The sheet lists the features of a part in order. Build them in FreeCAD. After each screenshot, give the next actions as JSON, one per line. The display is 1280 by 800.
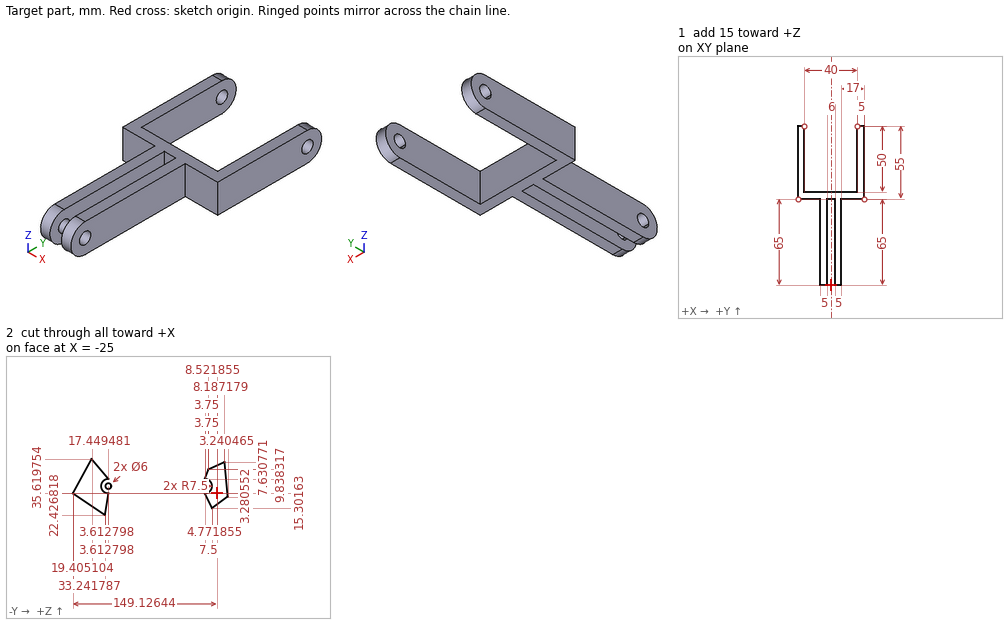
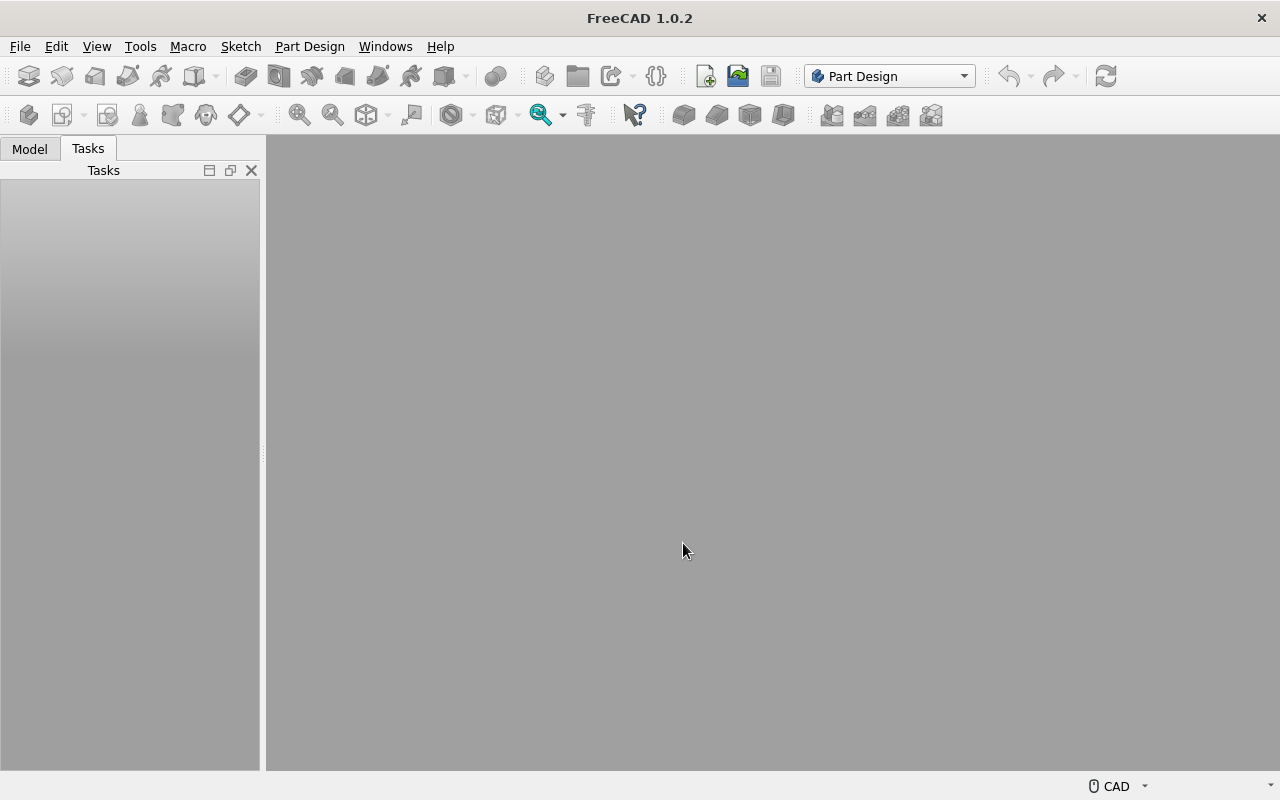
{"action": "key", "text": "ctrl+n"}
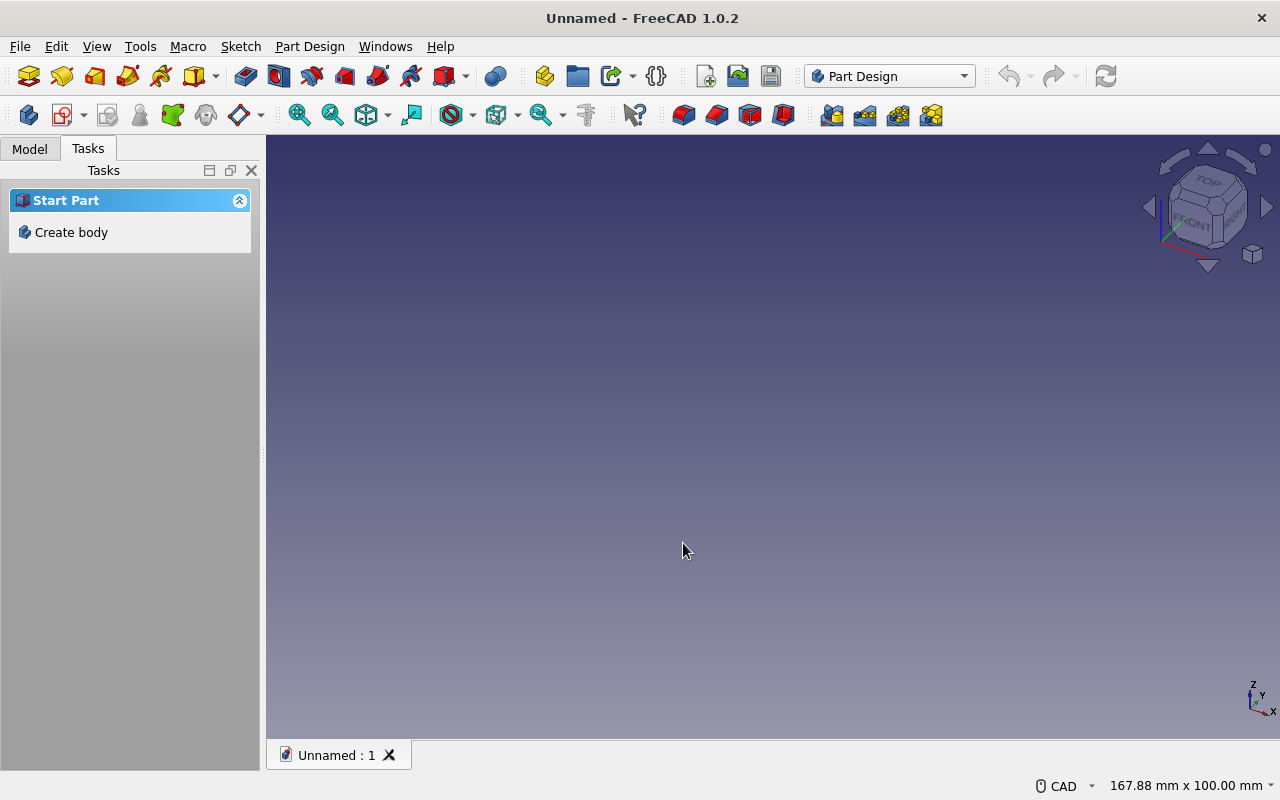
{"action": "left_click", "coordinate": [62, 116]}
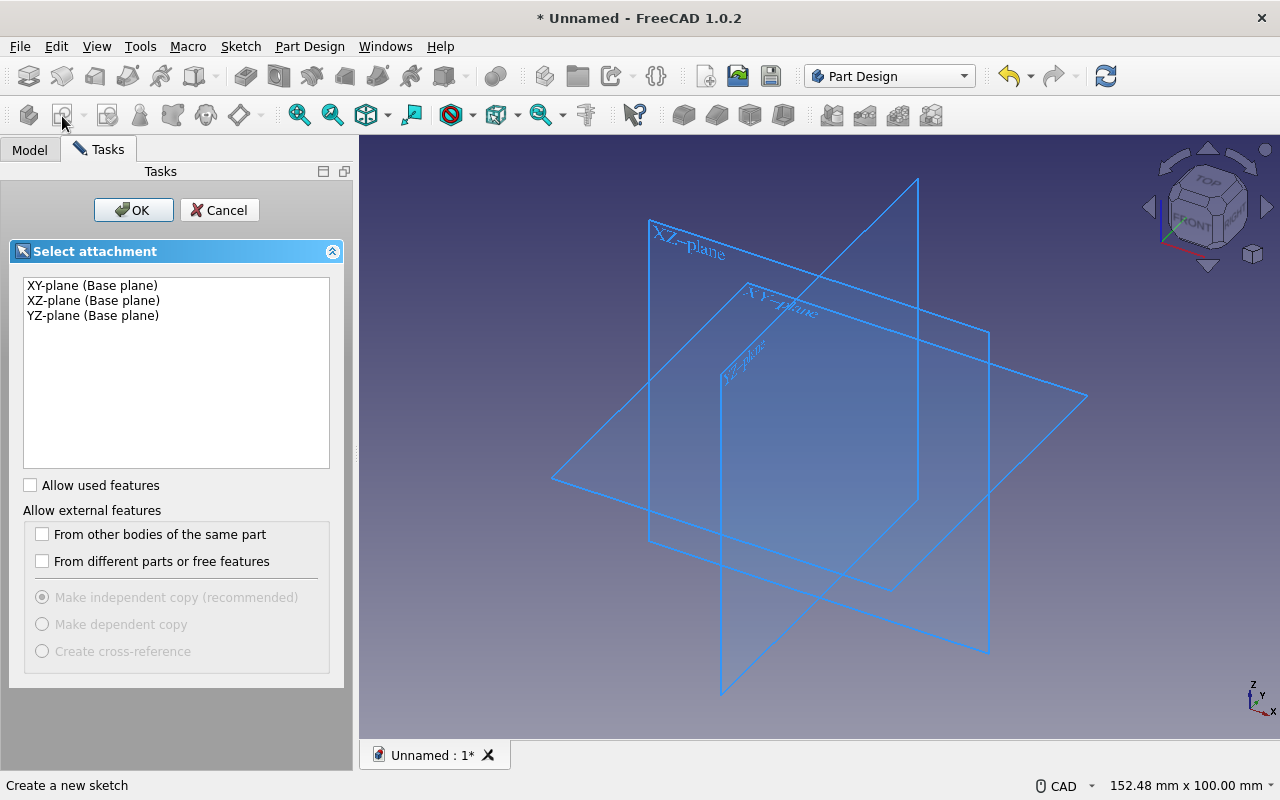
{"action": "left_click", "coordinate": [84, 286]}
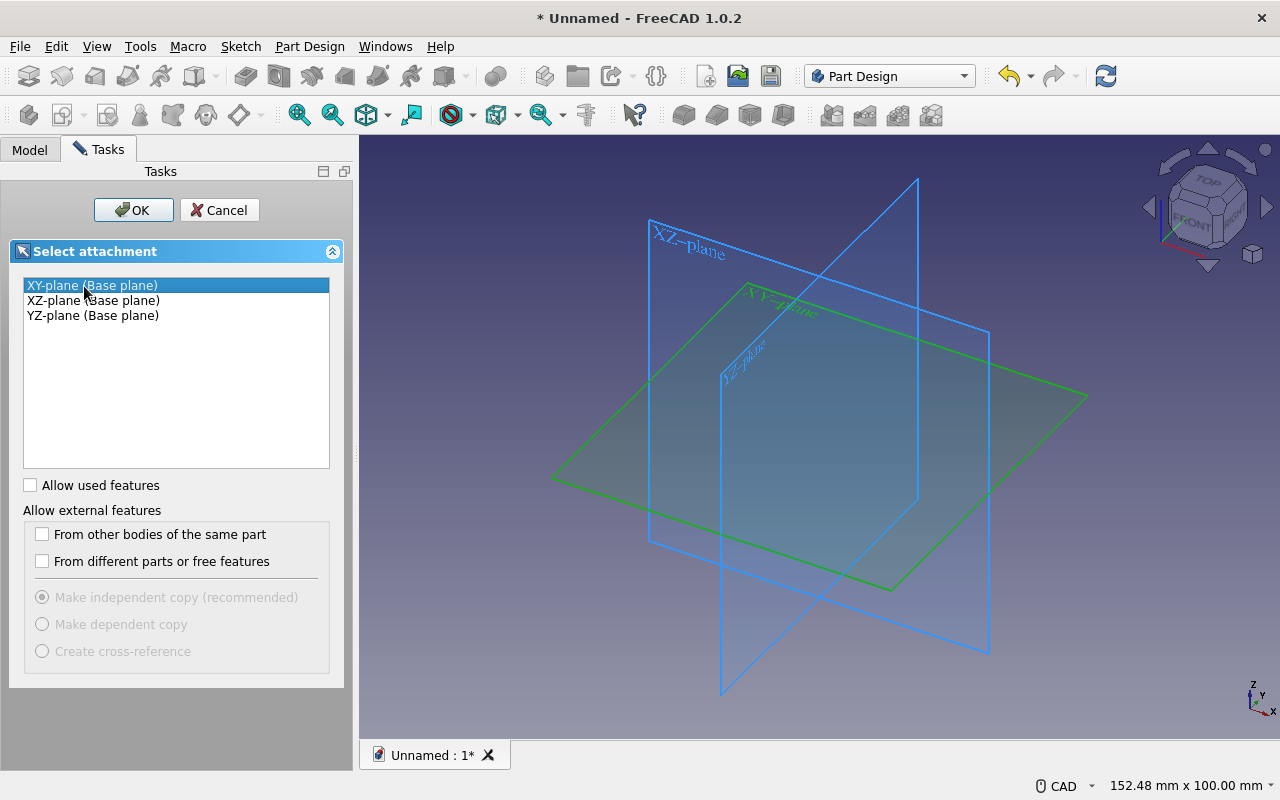
{"action": "left_click", "coordinate": [134, 210]}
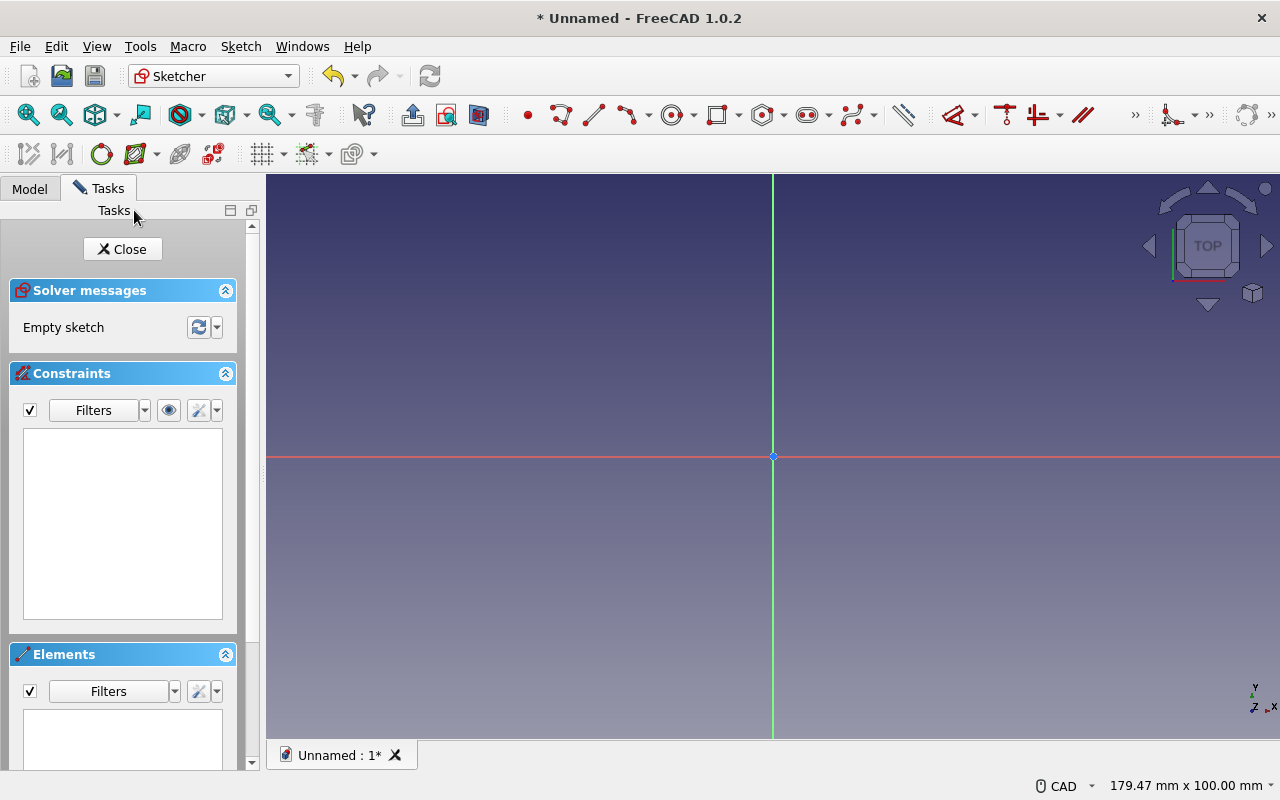
{"action": "scroll", "coordinate": [649, 711], "scroll_direction": "down", "scroll_amount": 4}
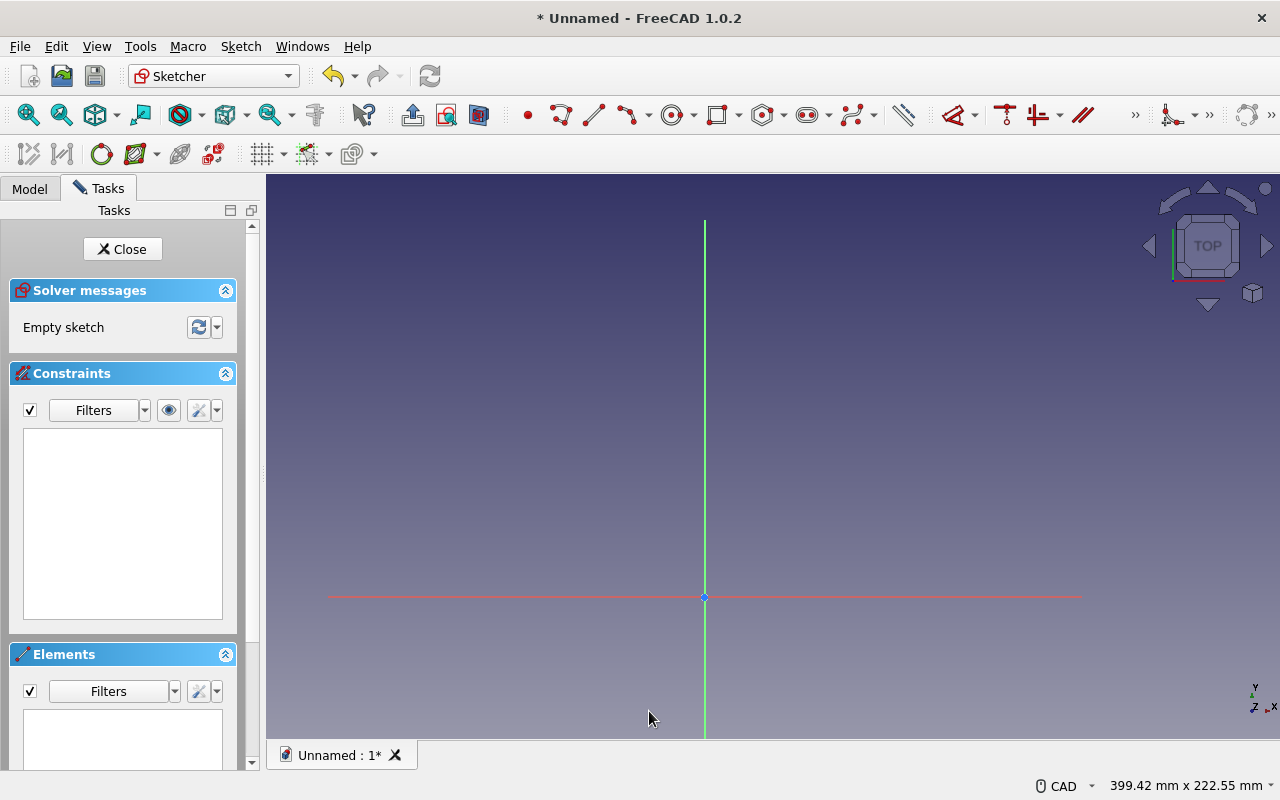
{"action": "key", "text": "g m"}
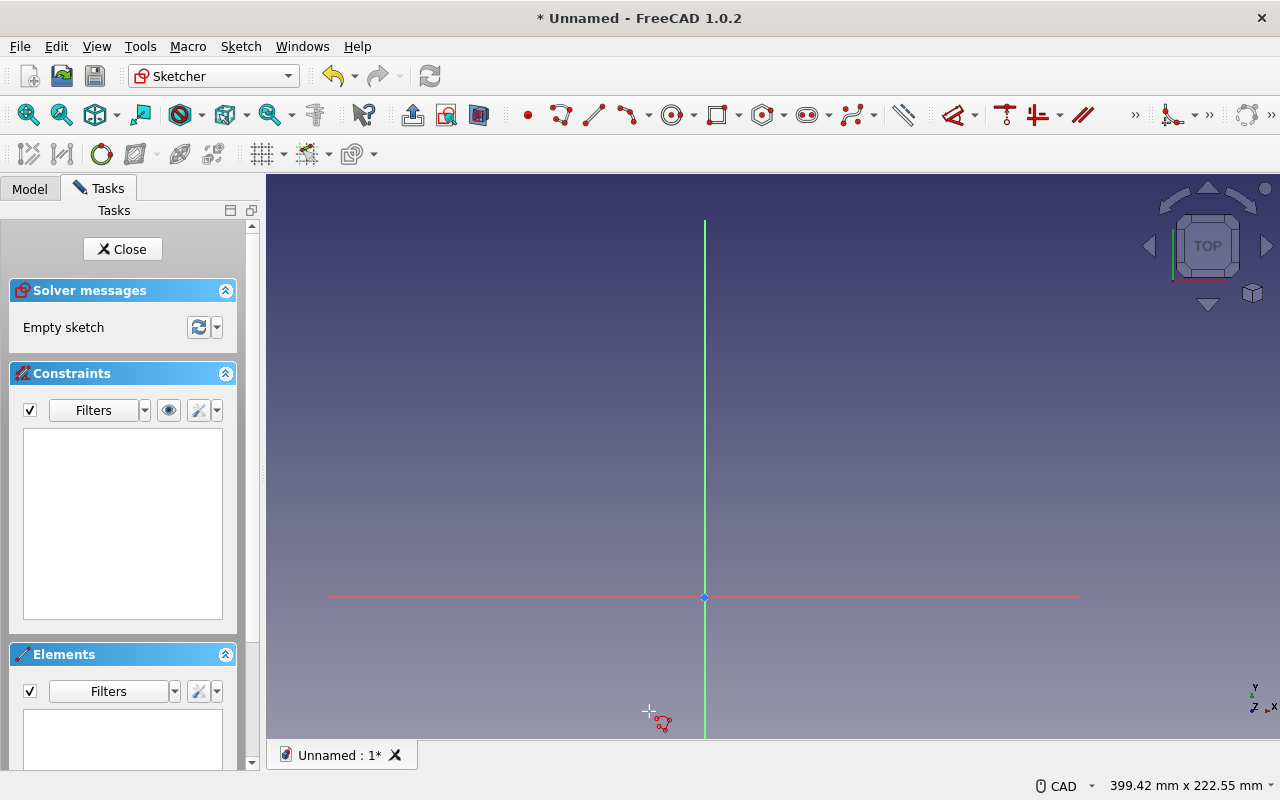
{"action": "scroll", "coordinate": [697, 597], "scroll_direction": "up", "scroll_amount": 4}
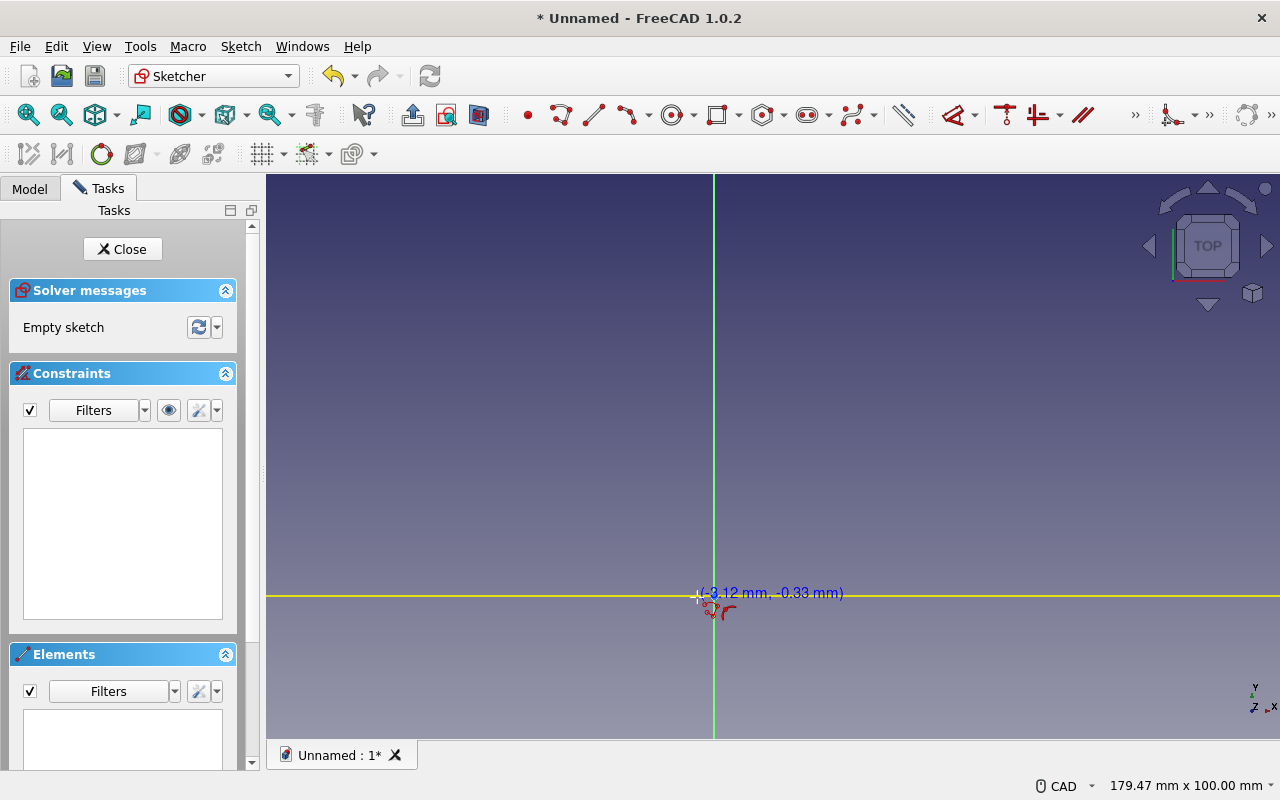
{"action": "left_click", "coordinate": [697, 596]}
{"action": "left_click", "coordinate": [697, 229]}
{"action": "left_click", "coordinate": [731, 229]}
{"action": "left_click", "coordinate": [731, 596]}
{"action": "left_click", "coordinate": [759, 587]}
{"action": "left_click", "coordinate": [759, 229]}
{"action": "left_click", "coordinate": [855, 229]}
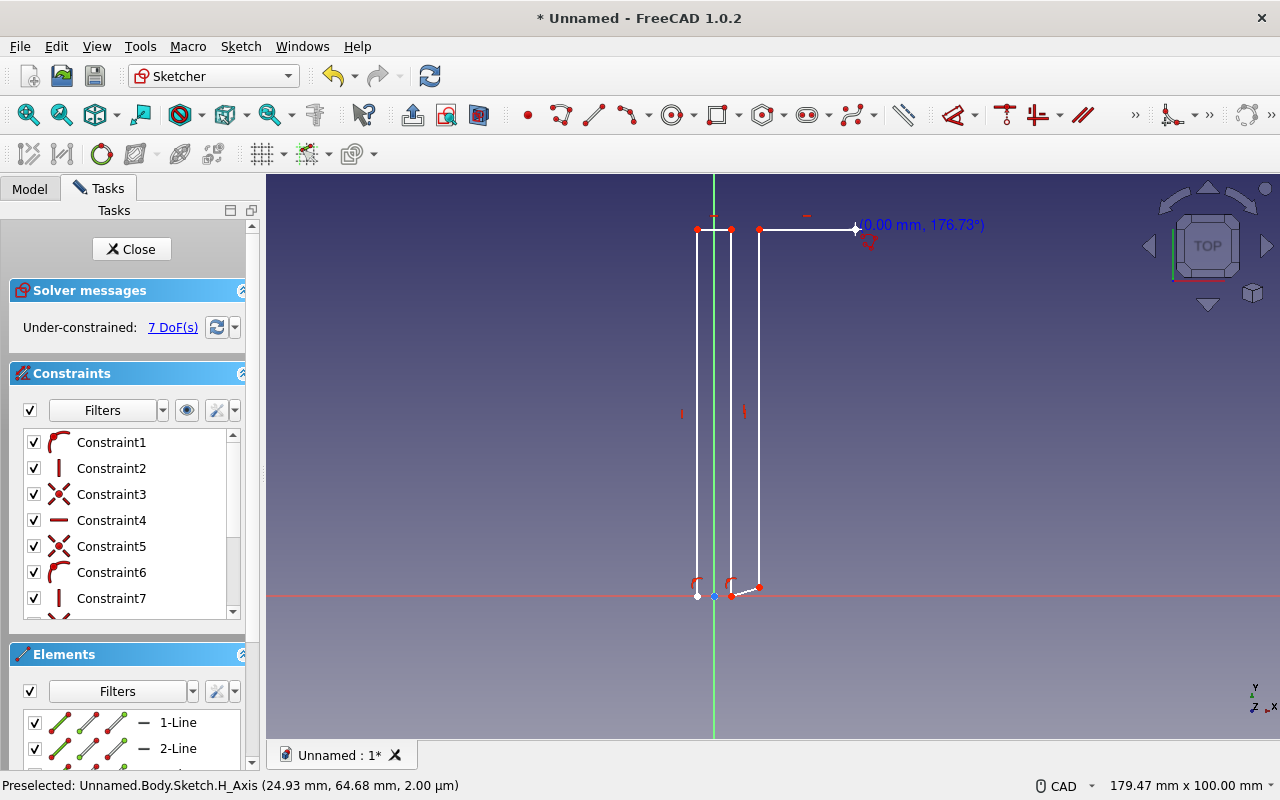
{"action": "scroll", "coordinate": [693, 699], "scroll_direction": "down", "scroll_amount": 3}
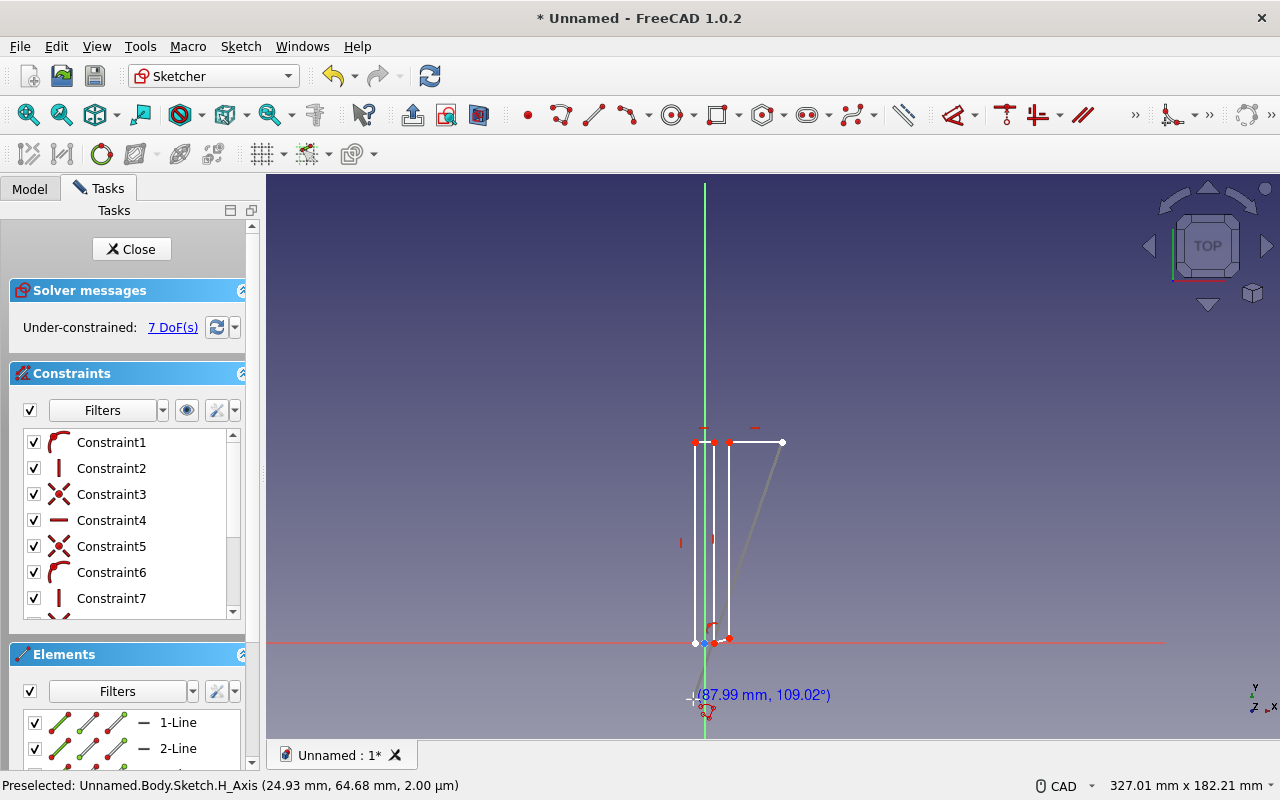
{"action": "left_click", "coordinate": [782, 271]}
{"action": "left_click", "coordinate": [767, 271]}
{"action": "left_click", "coordinate": [767, 426]}
{"action": "left_click", "coordinate": [643, 426]}
{"action": "left_click", "coordinate": [643, 271]}
{"action": "left_click", "coordinate": [627, 271]}
{"action": "left_click", "coordinate": [627, 442]}
{"action": "left_click", "coordinate": [680, 442]}
{"action": "left_click", "coordinate": [680, 634]}